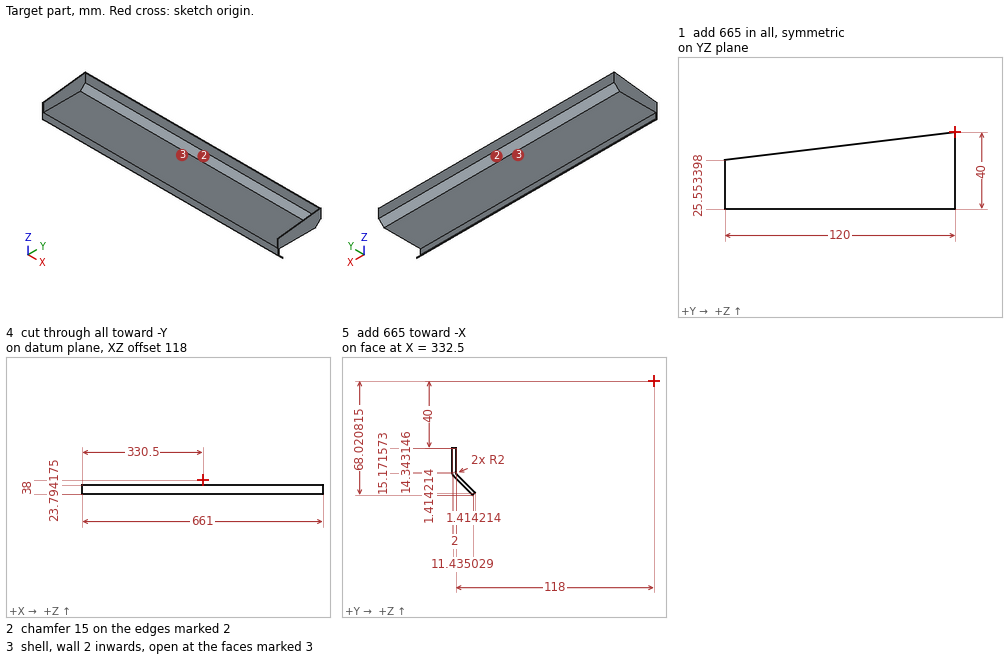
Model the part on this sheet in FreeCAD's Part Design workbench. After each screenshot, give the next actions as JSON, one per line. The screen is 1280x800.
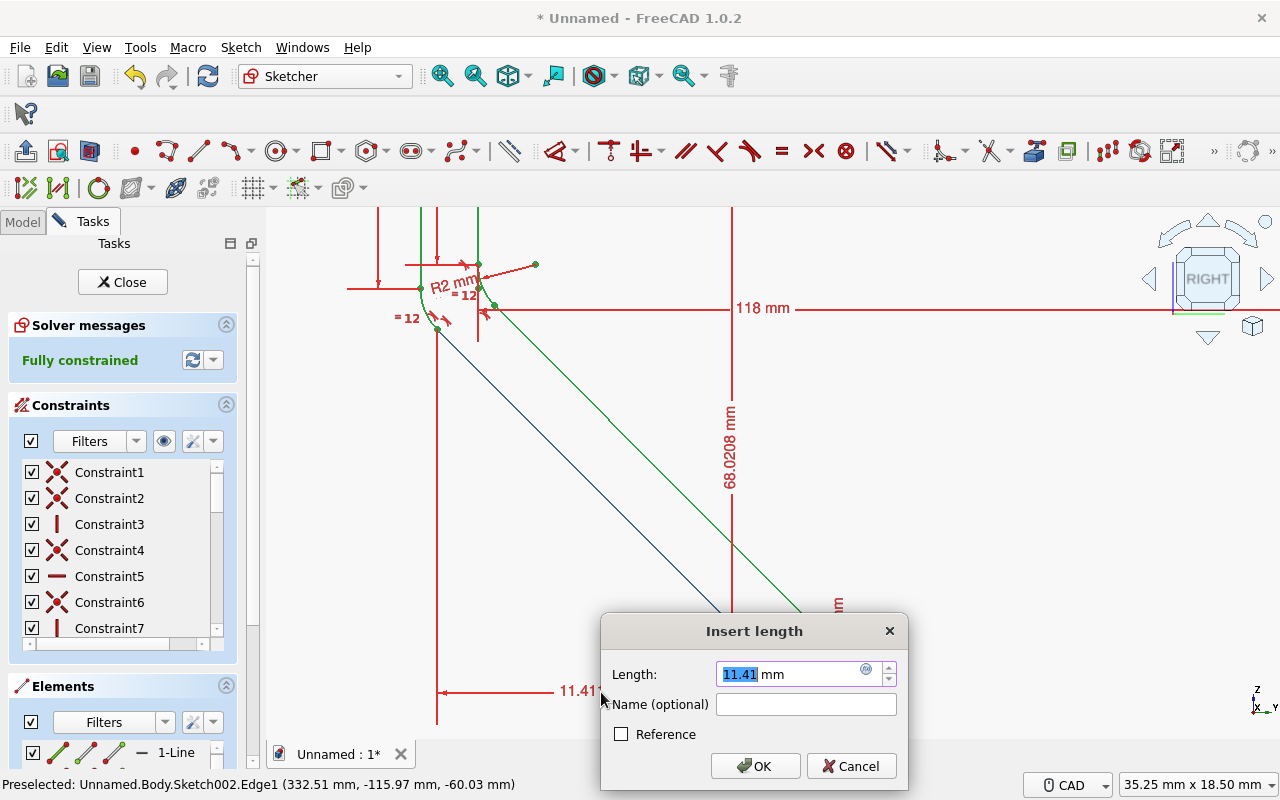
{"action": "type", "text": "11.435029"}
{"action": "key", "text": "Return"}
{"action": "key", "text": "Escape"}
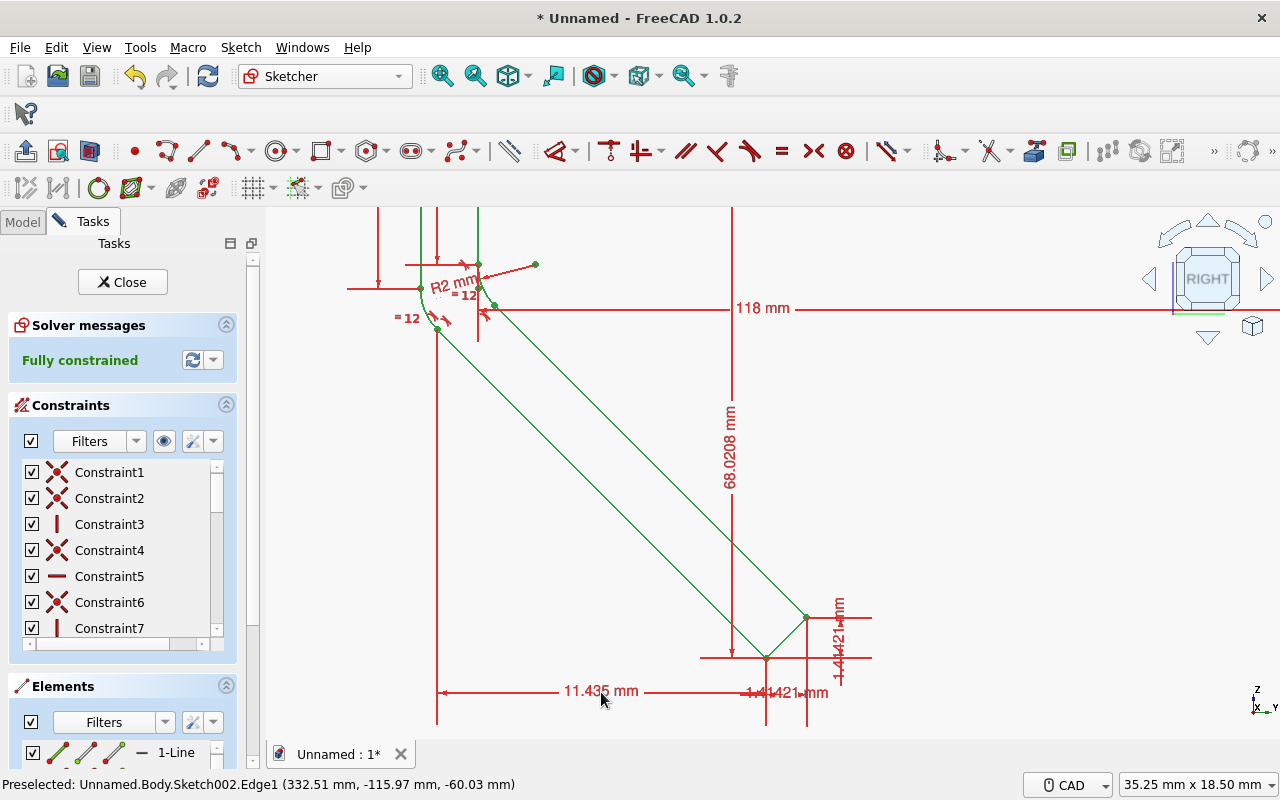
{"action": "left_click", "coordinate": [123, 282]}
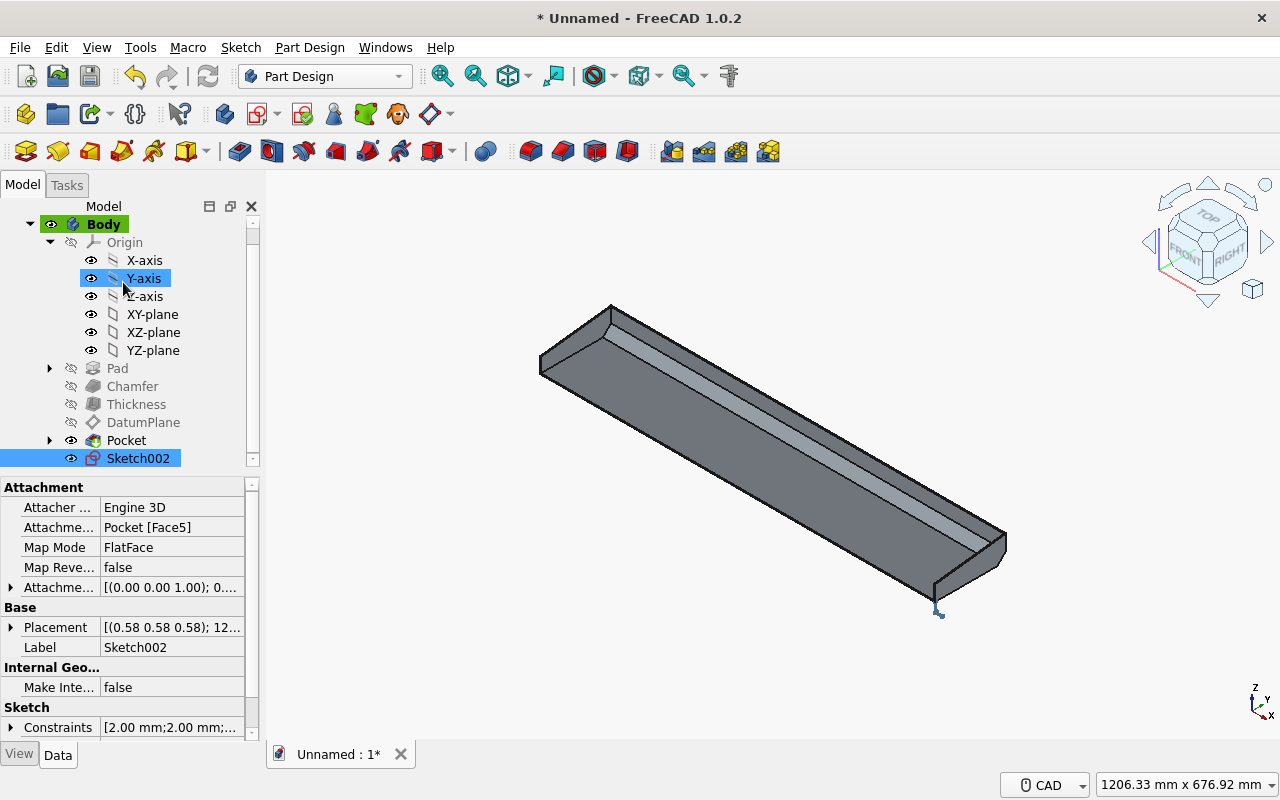
{"action": "left_click", "coordinate": [26, 152]}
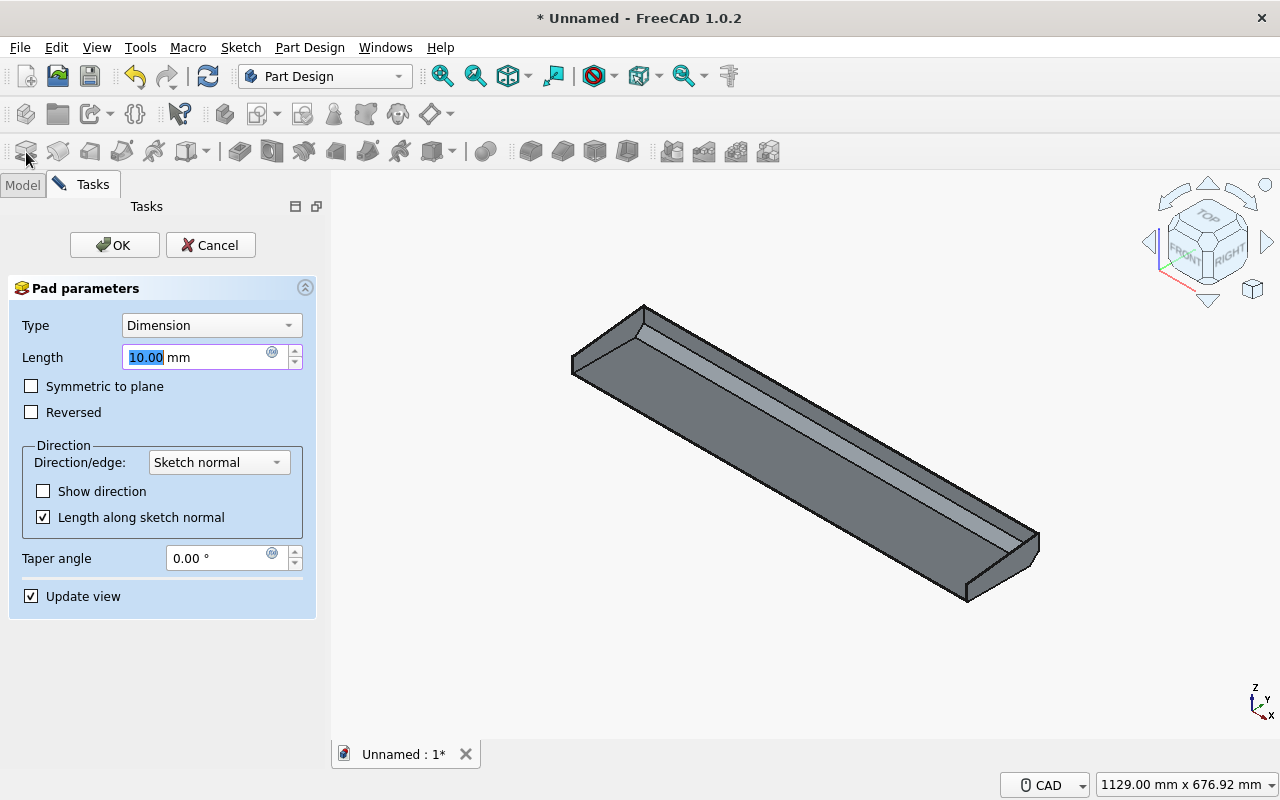
{"action": "type", "text": "665"}
{"action": "key", "text": "Tab"}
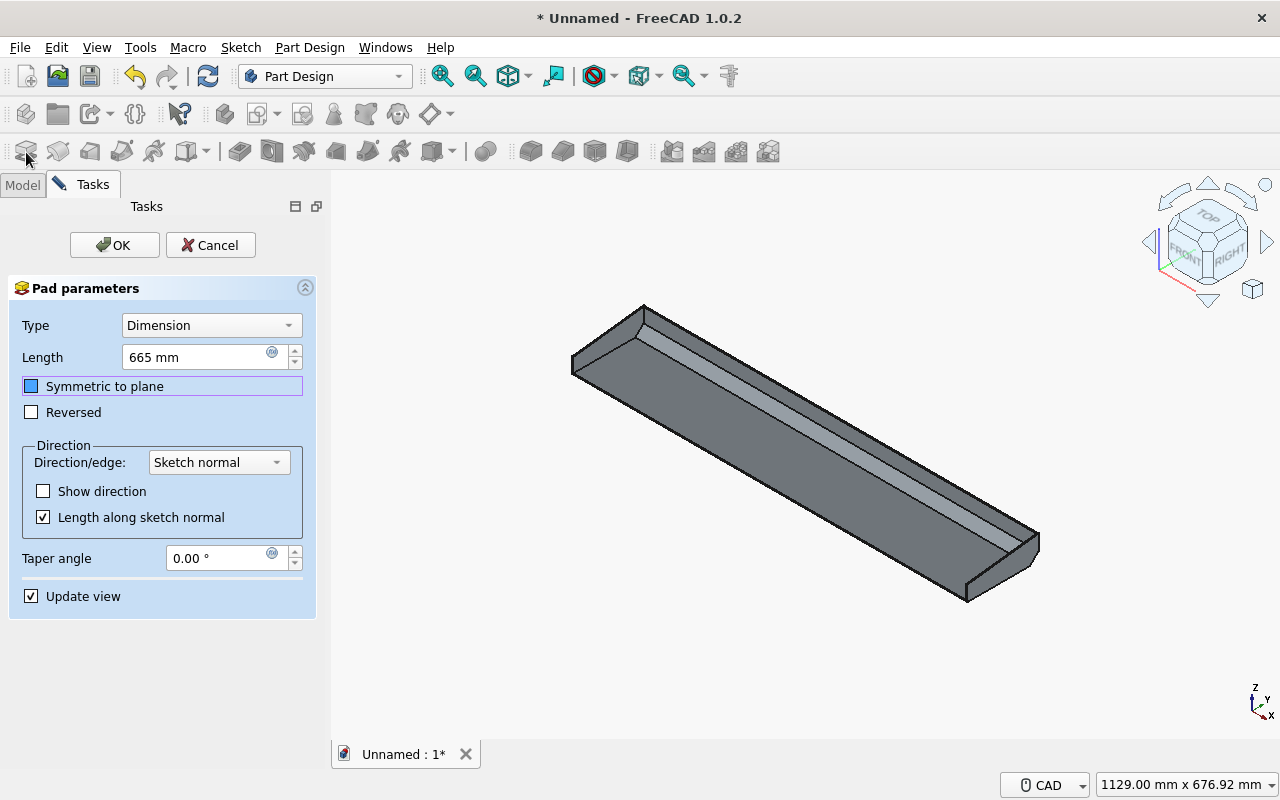
{"action": "left_click", "coordinate": [30, 412]}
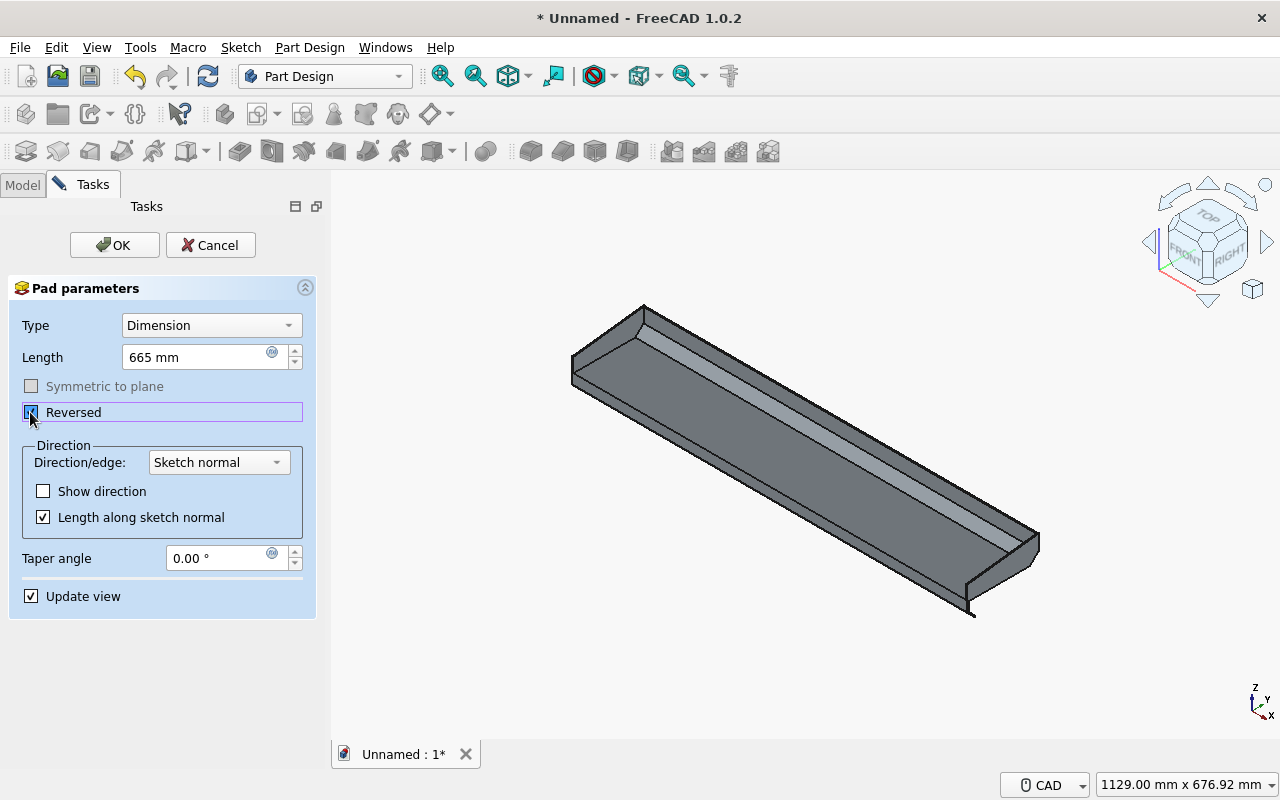
{"action": "left_click", "coordinate": [115, 245]}